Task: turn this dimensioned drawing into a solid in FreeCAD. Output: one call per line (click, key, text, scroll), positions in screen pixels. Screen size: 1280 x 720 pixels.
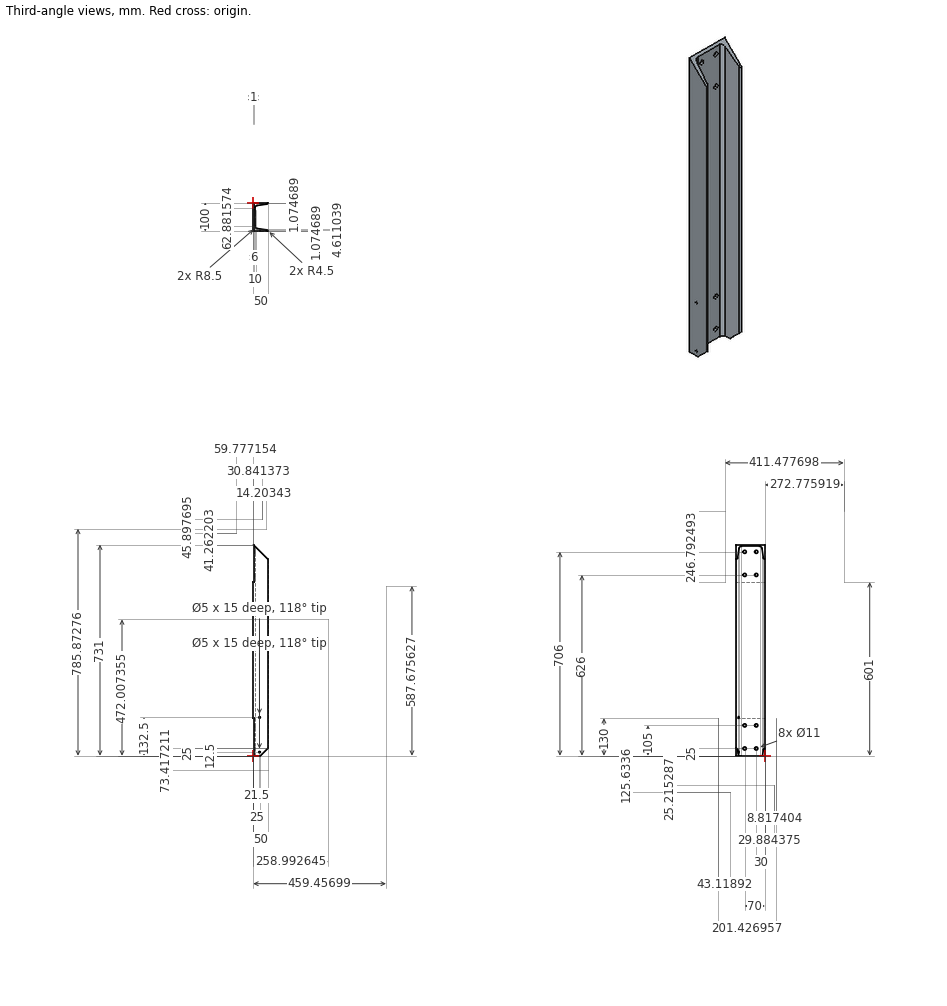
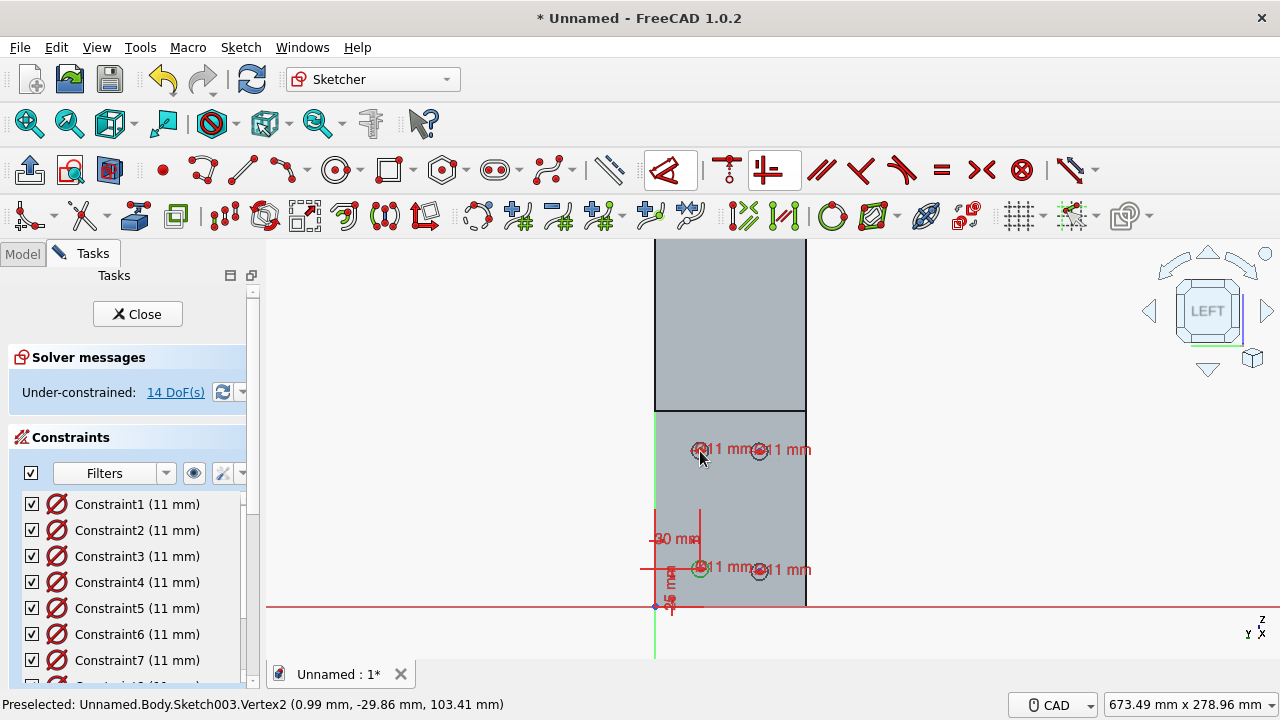
key(l)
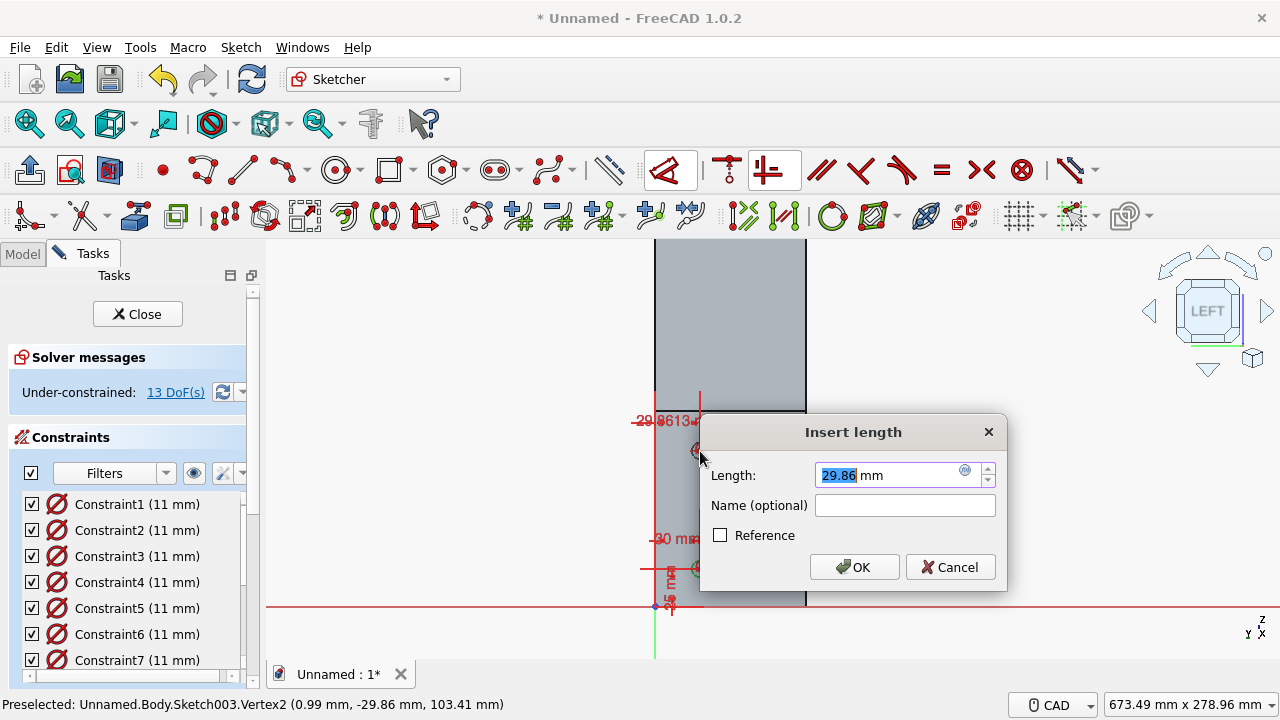
text(30)
key(Return)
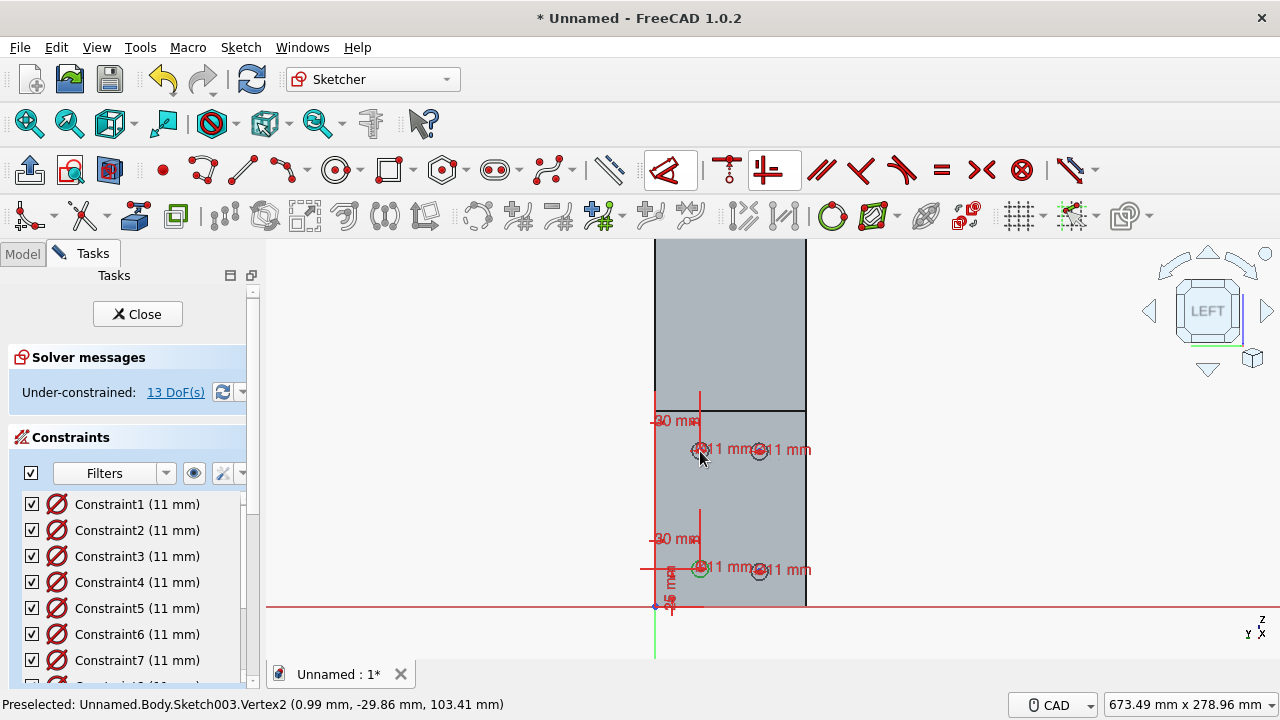
click(760, 572)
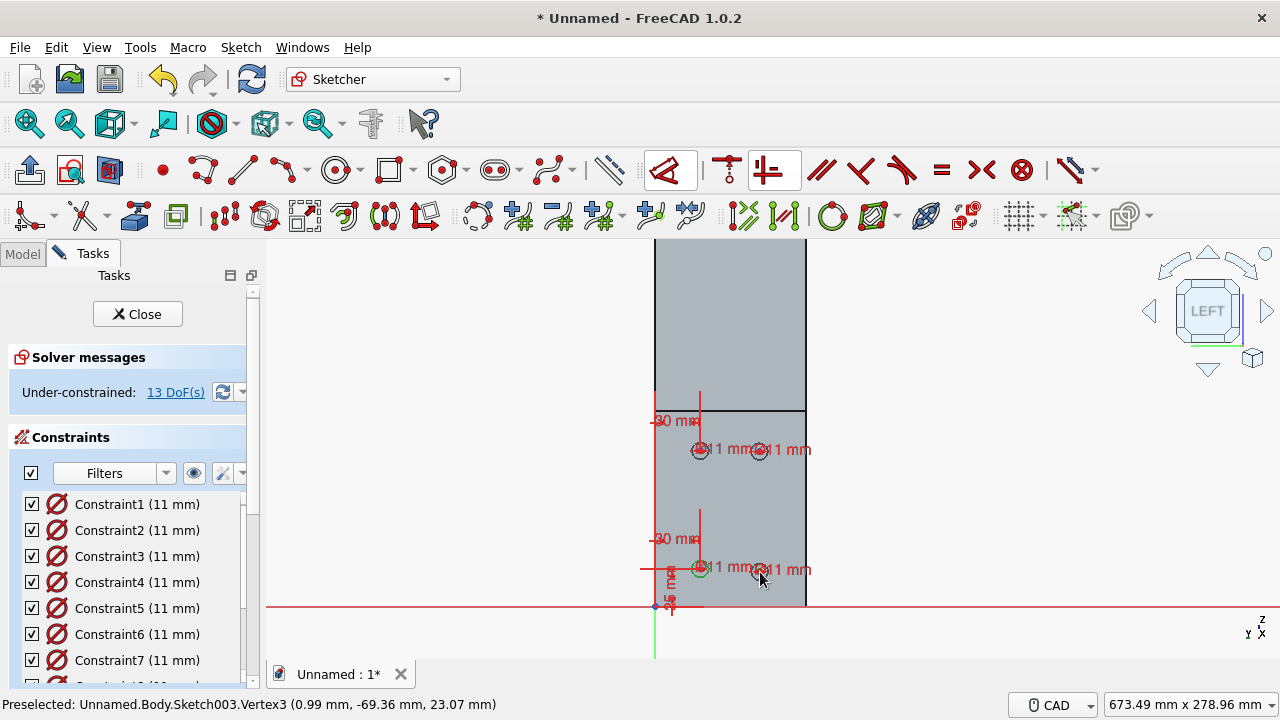
key(l)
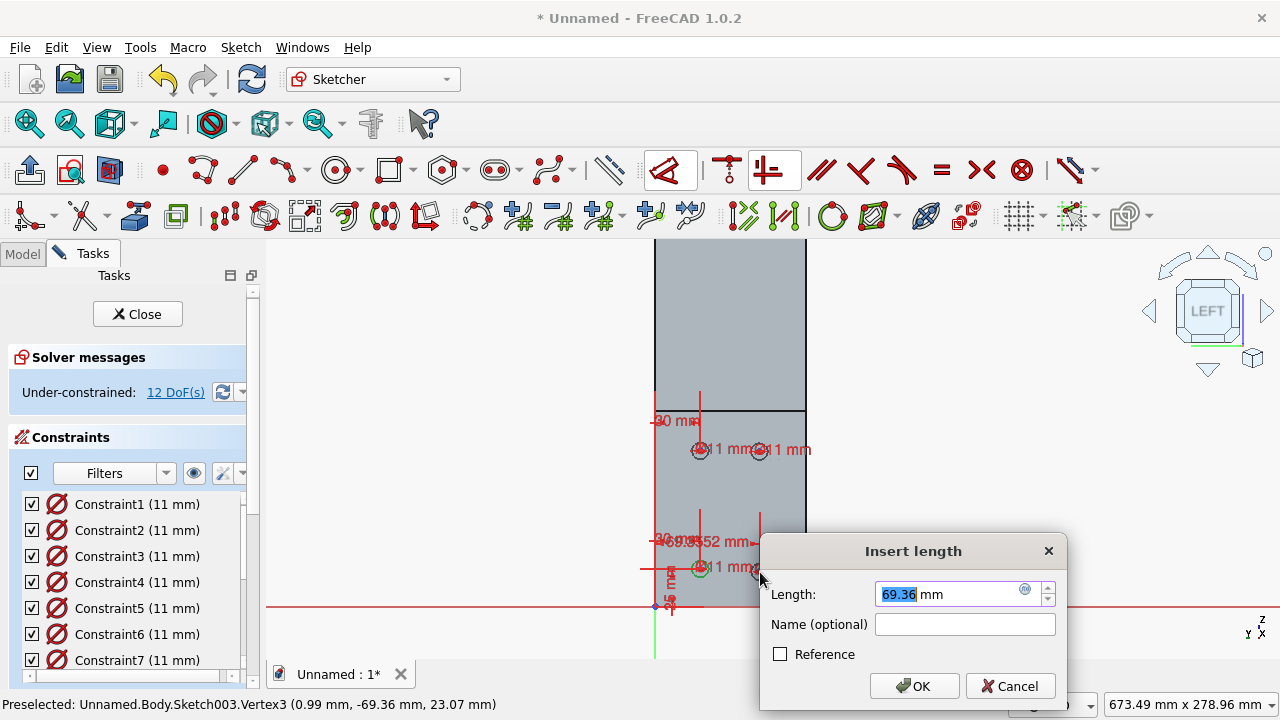
text(70)
key(Return)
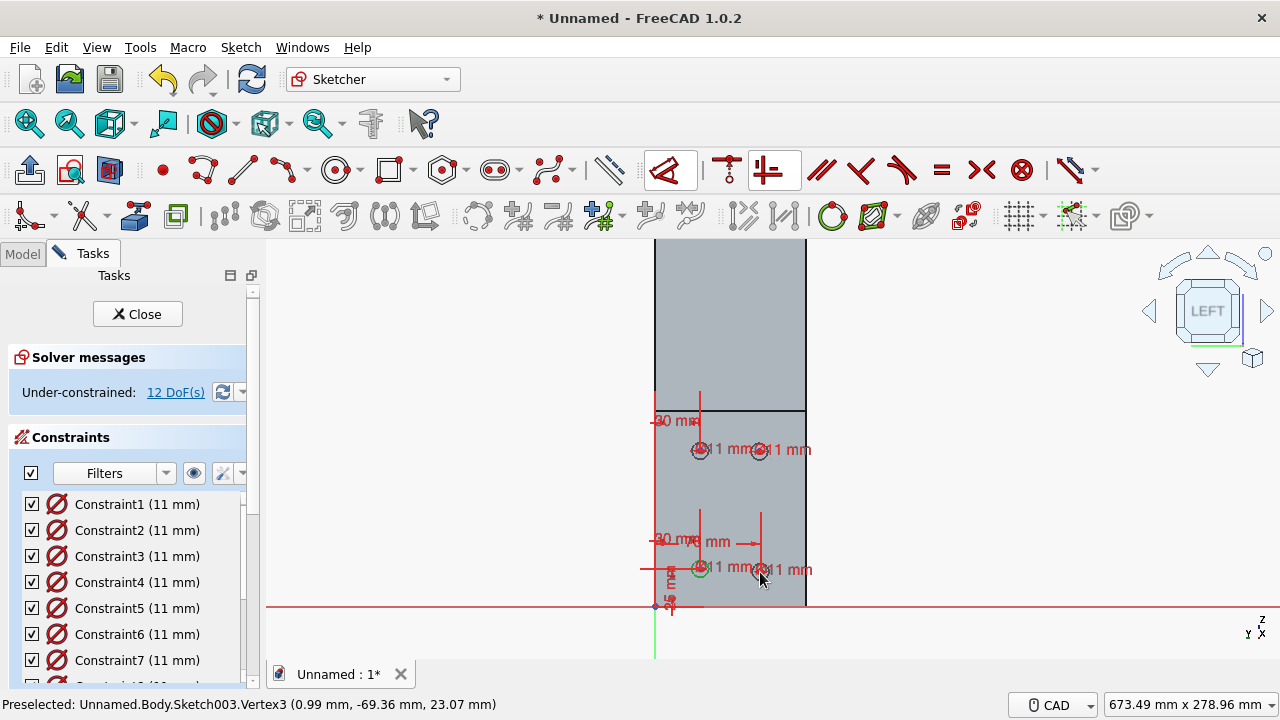
click(761, 572)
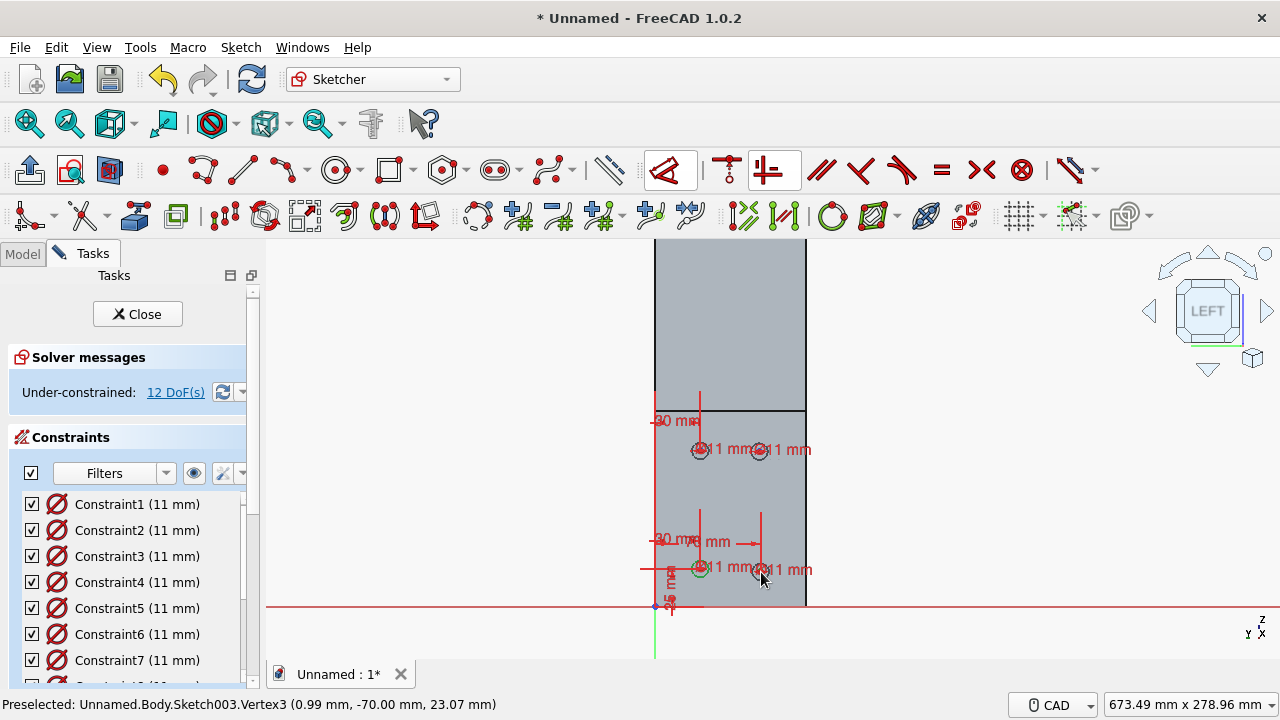
key(i)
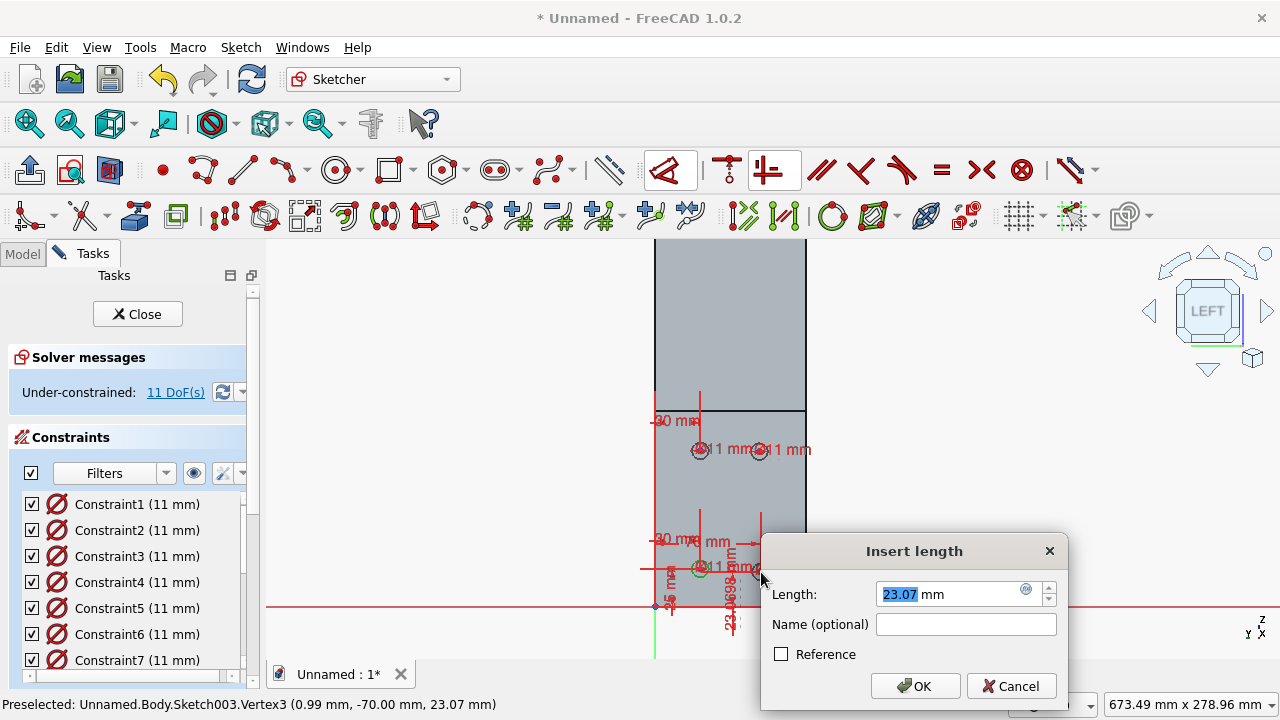
text(25)
key(Return)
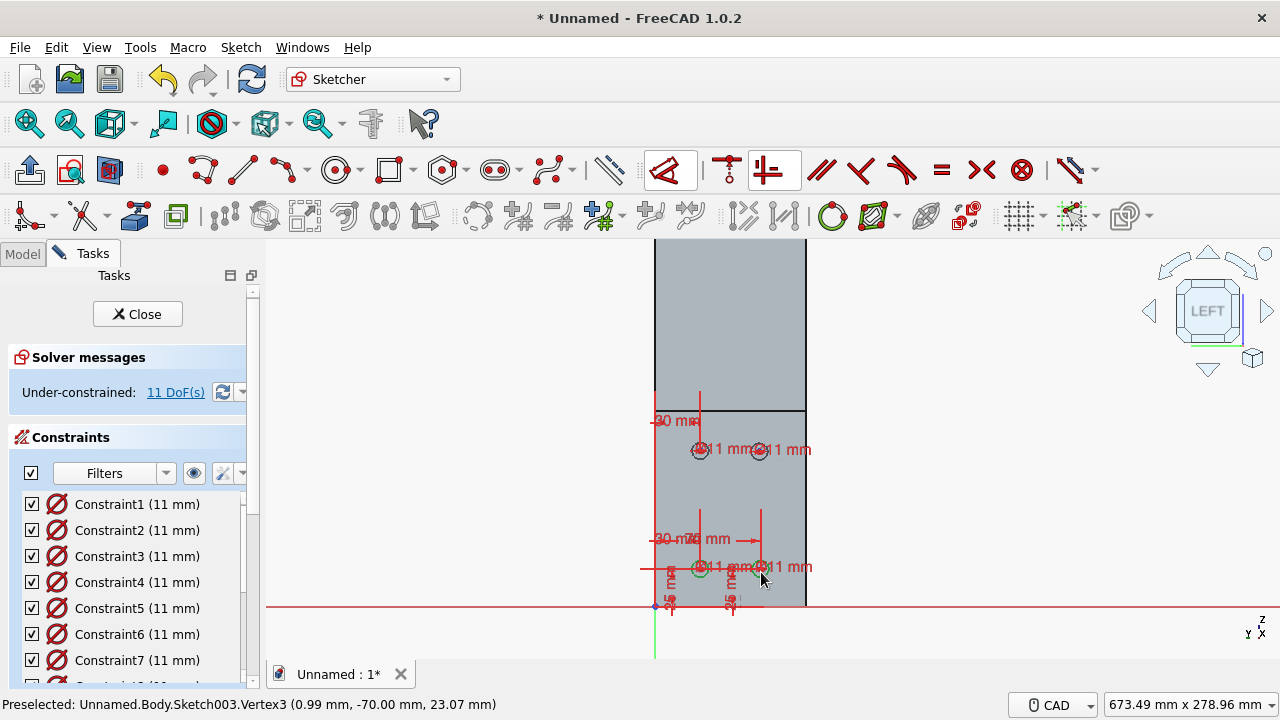
click(759, 452)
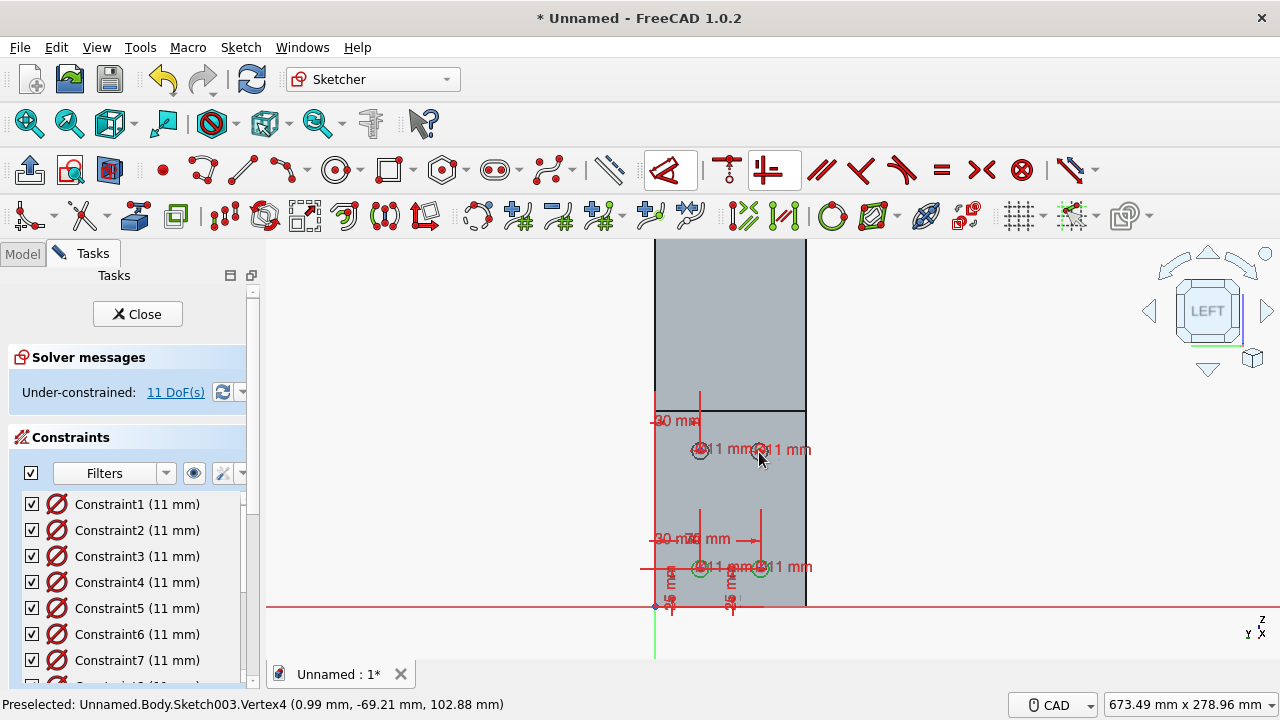
key(l)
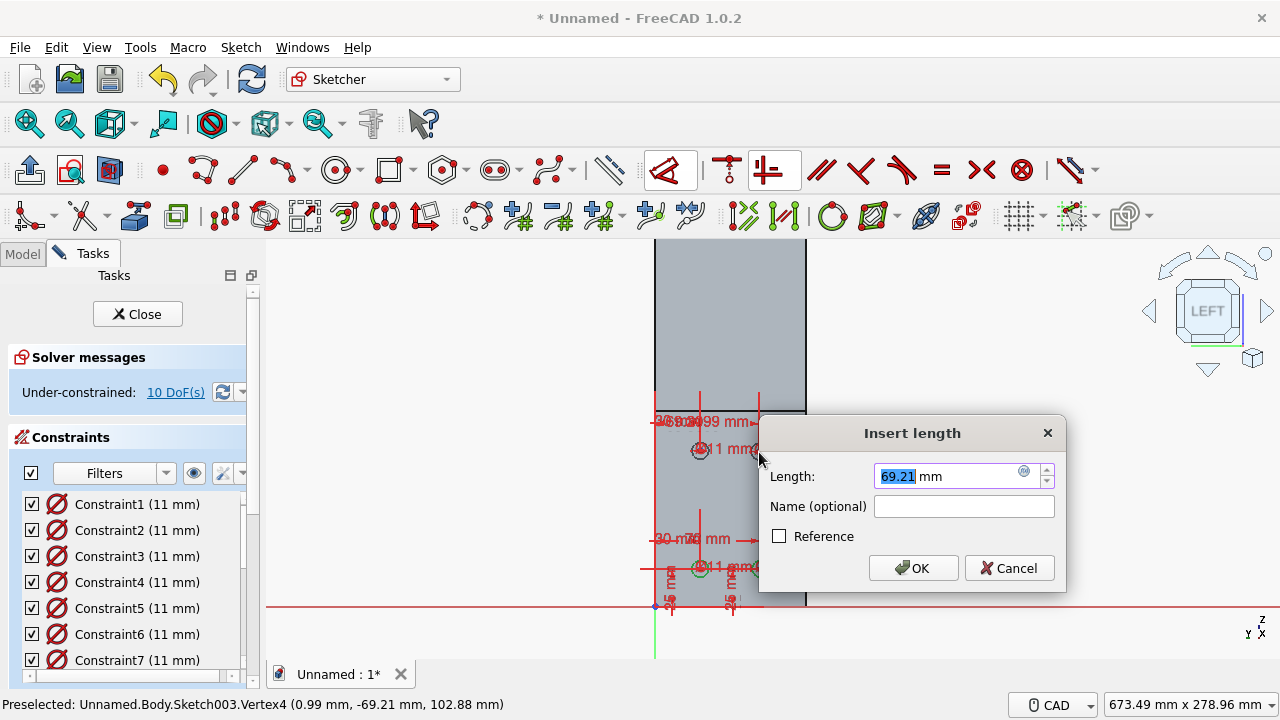
text(70)
key(Return)